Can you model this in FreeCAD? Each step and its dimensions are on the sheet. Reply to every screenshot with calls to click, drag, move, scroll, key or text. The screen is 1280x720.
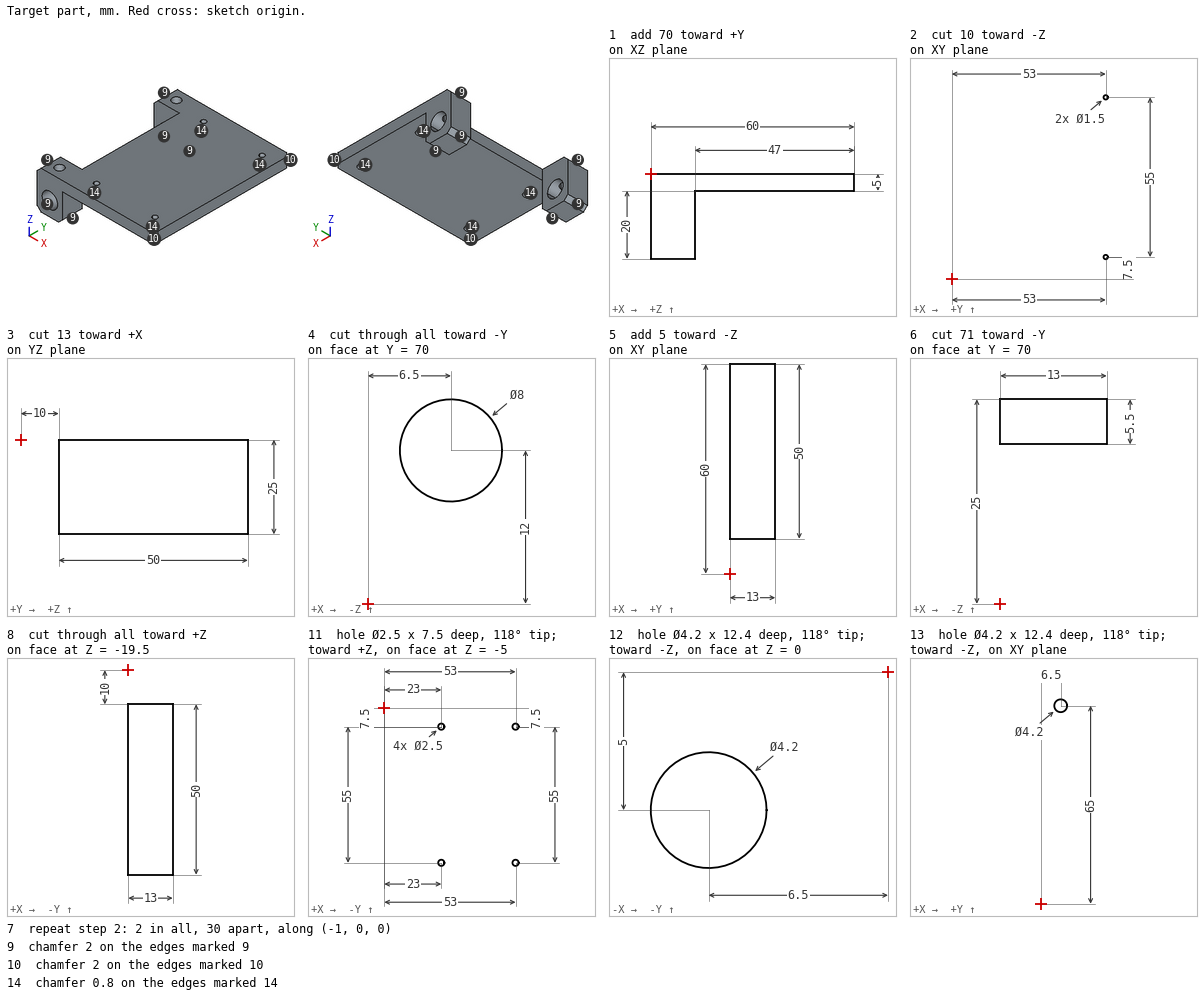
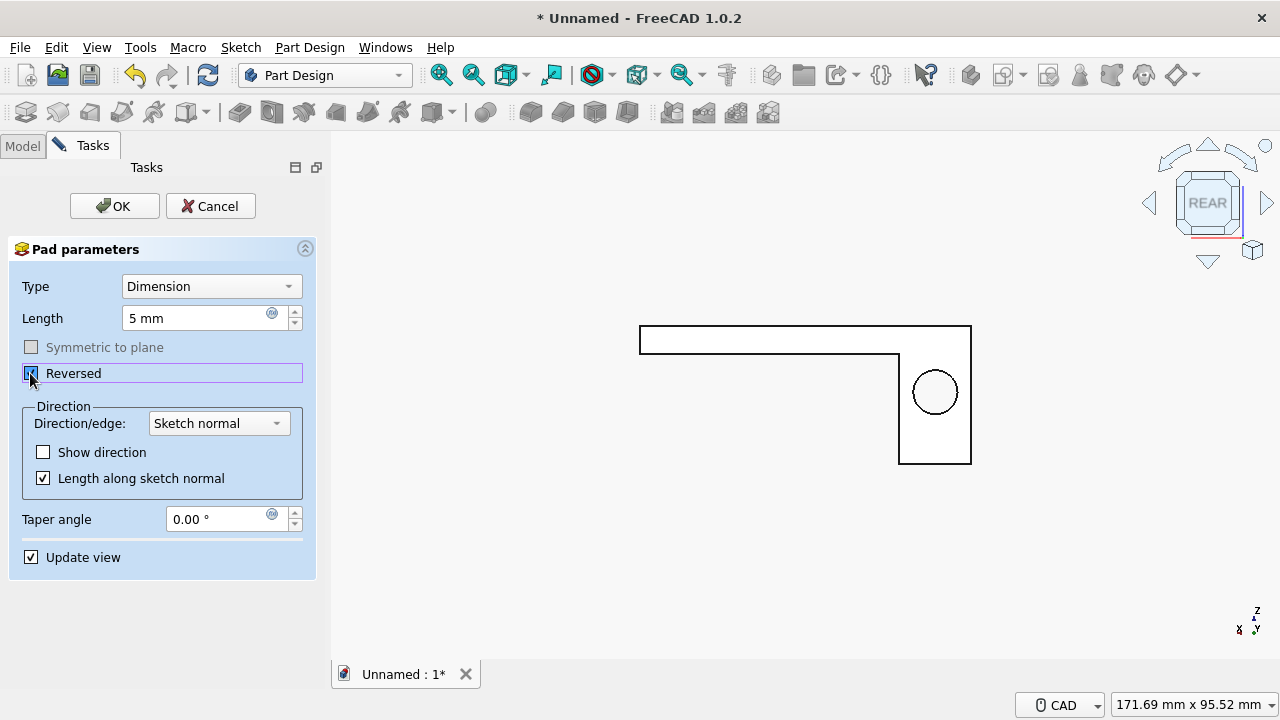
click(115, 206)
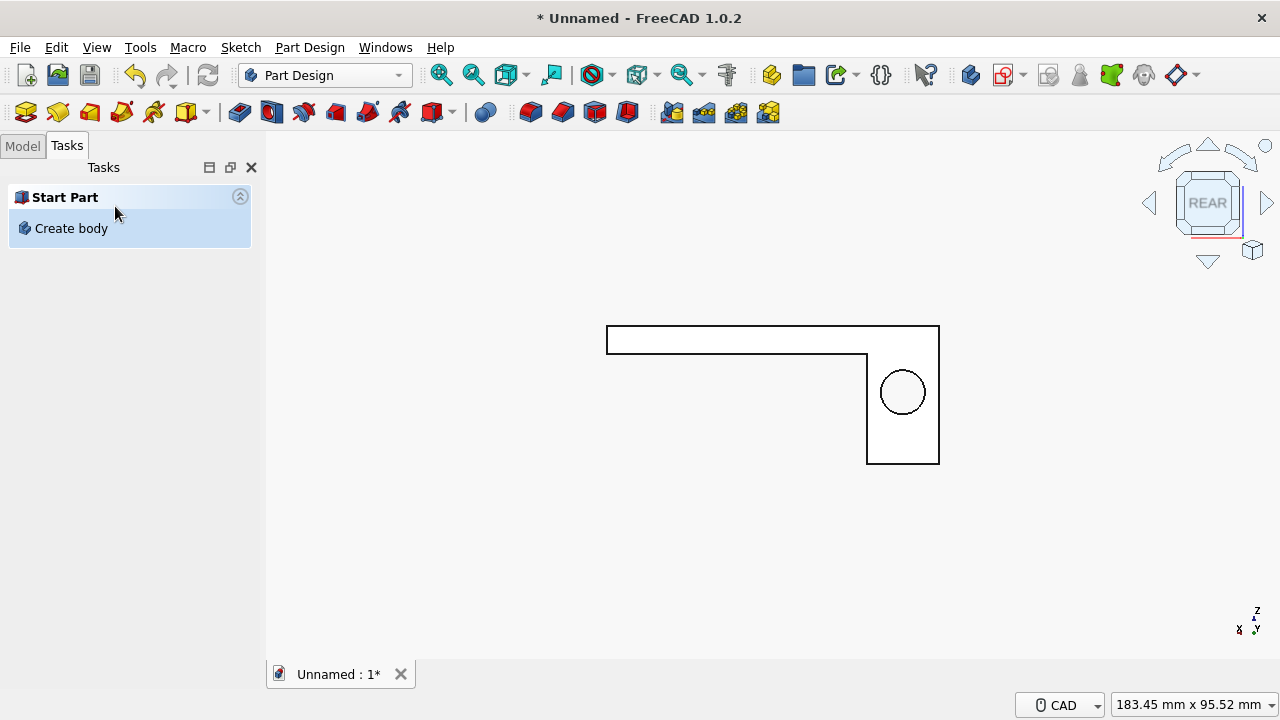
key(v)
key(f)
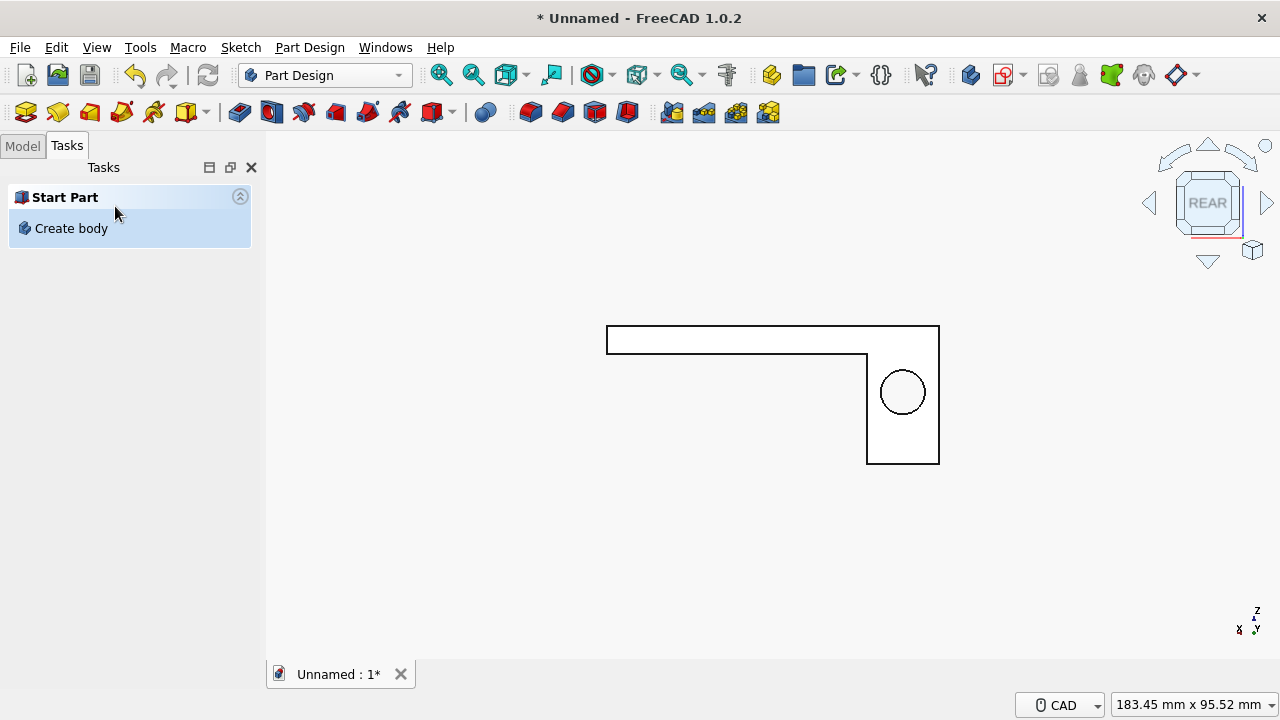
click(915, 433)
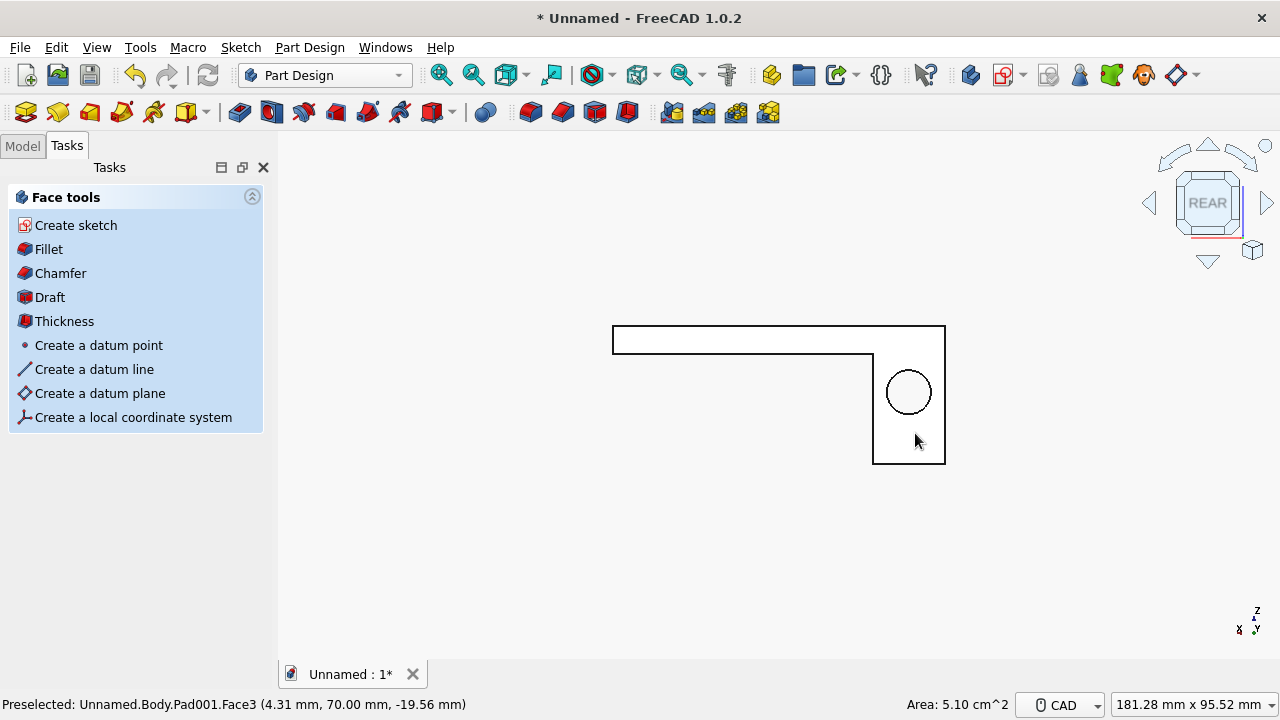
click(1004, 76)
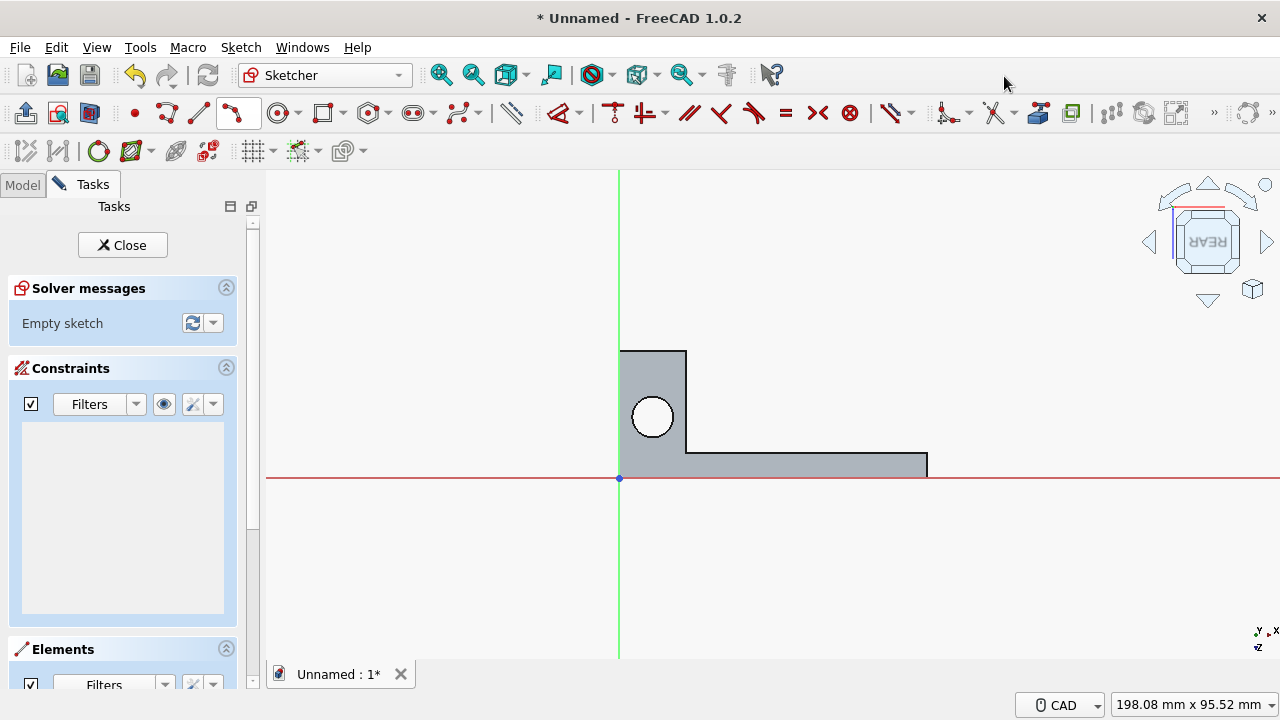
scroll(610, 414, up, 4)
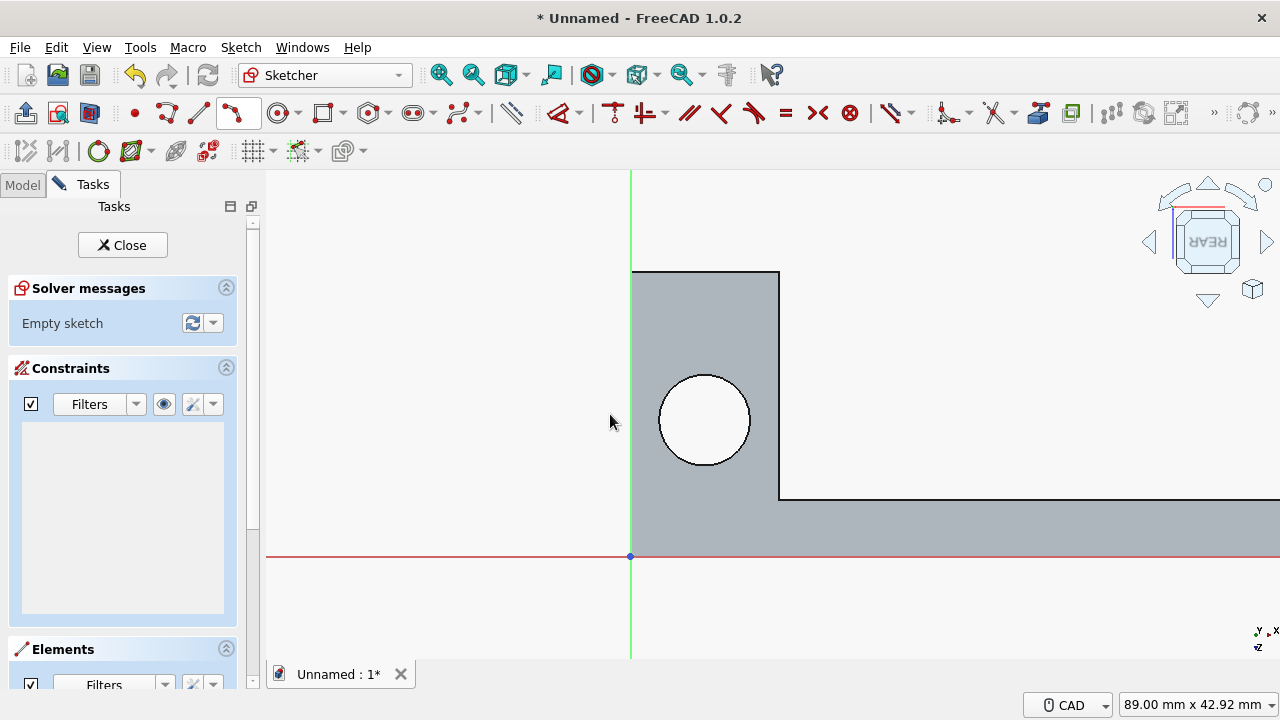
click(324, 114)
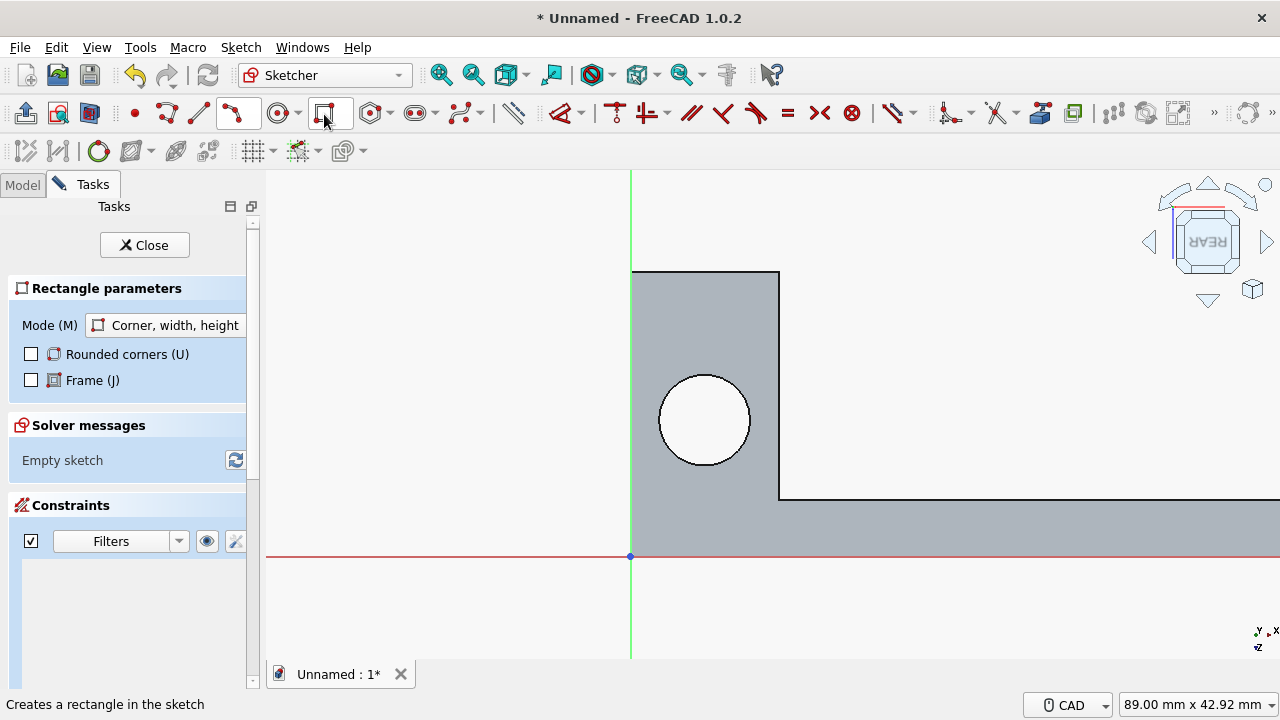
click(631, 272)
move(779, 335)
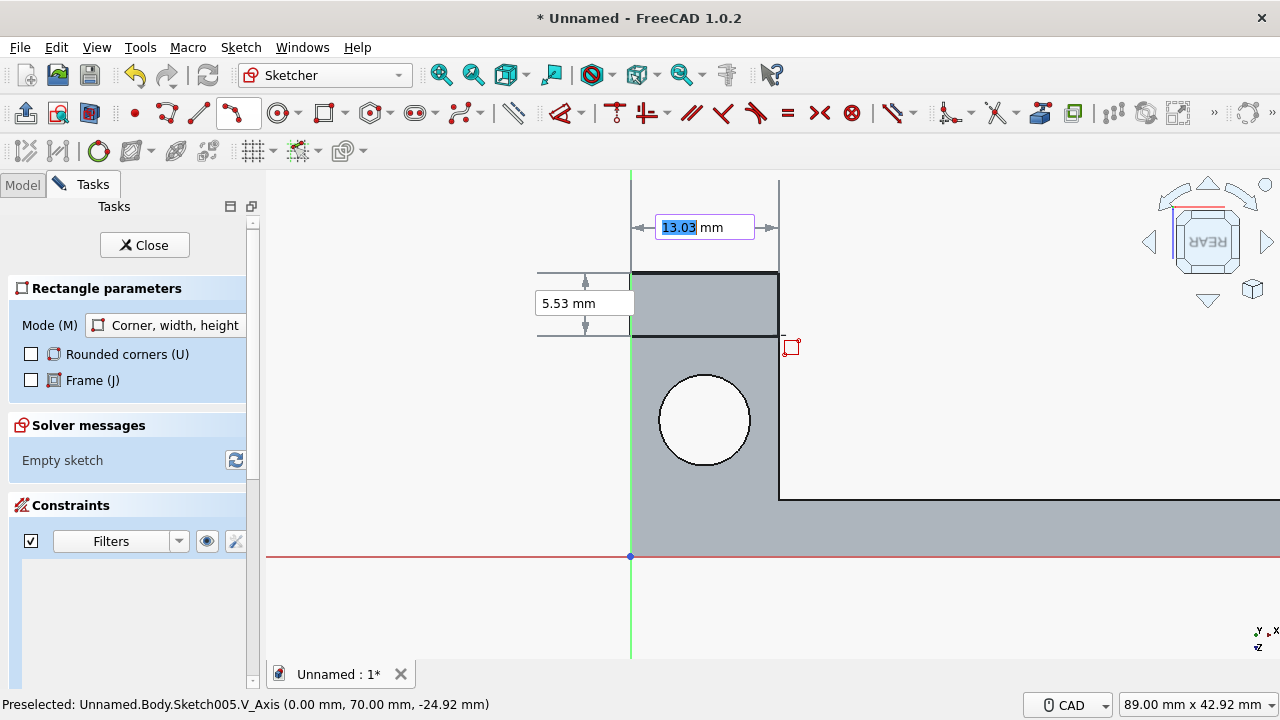
text(13)
key(Tab)
text(5.5)
key(Return)
key(Escape)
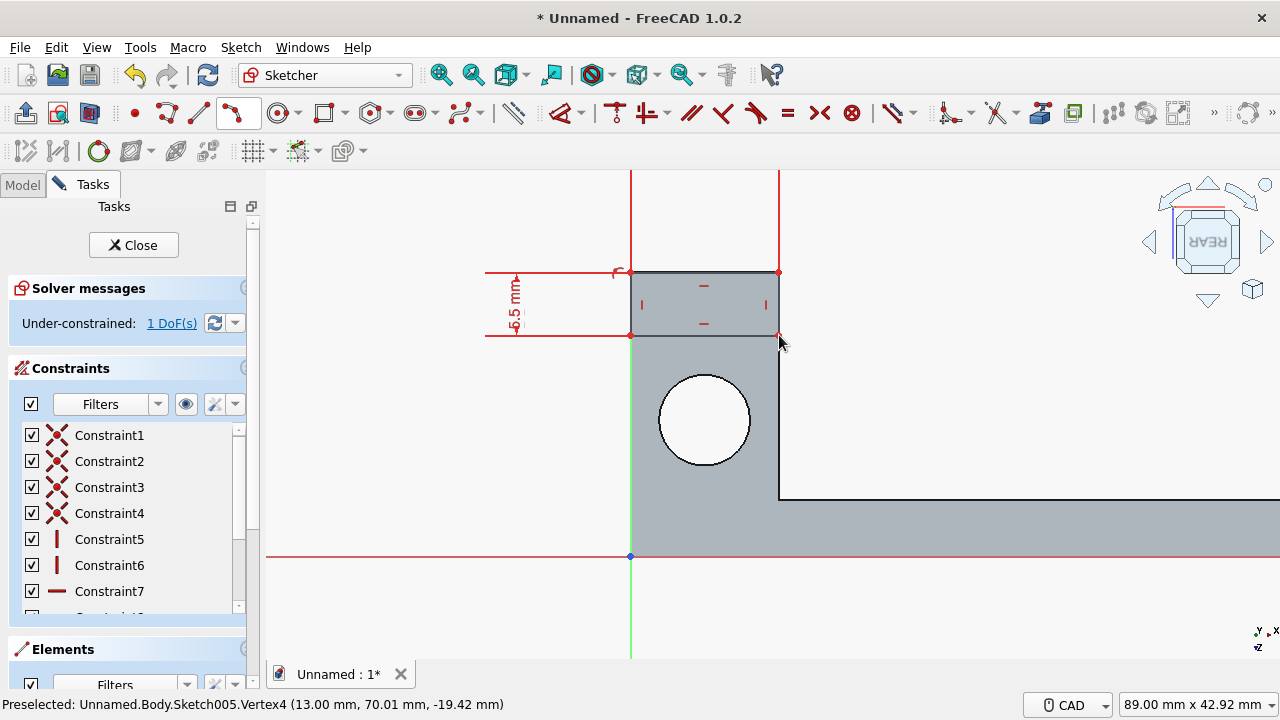
key(d)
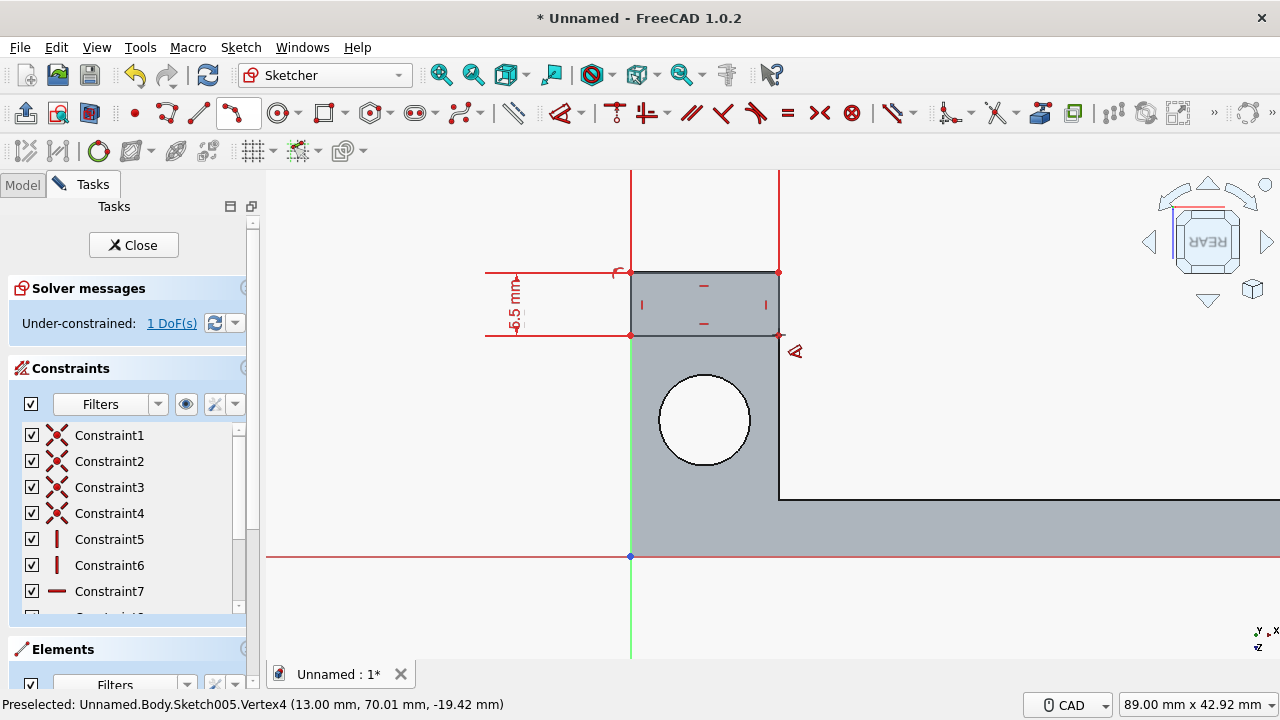
click(631, 273)
click(597, 415)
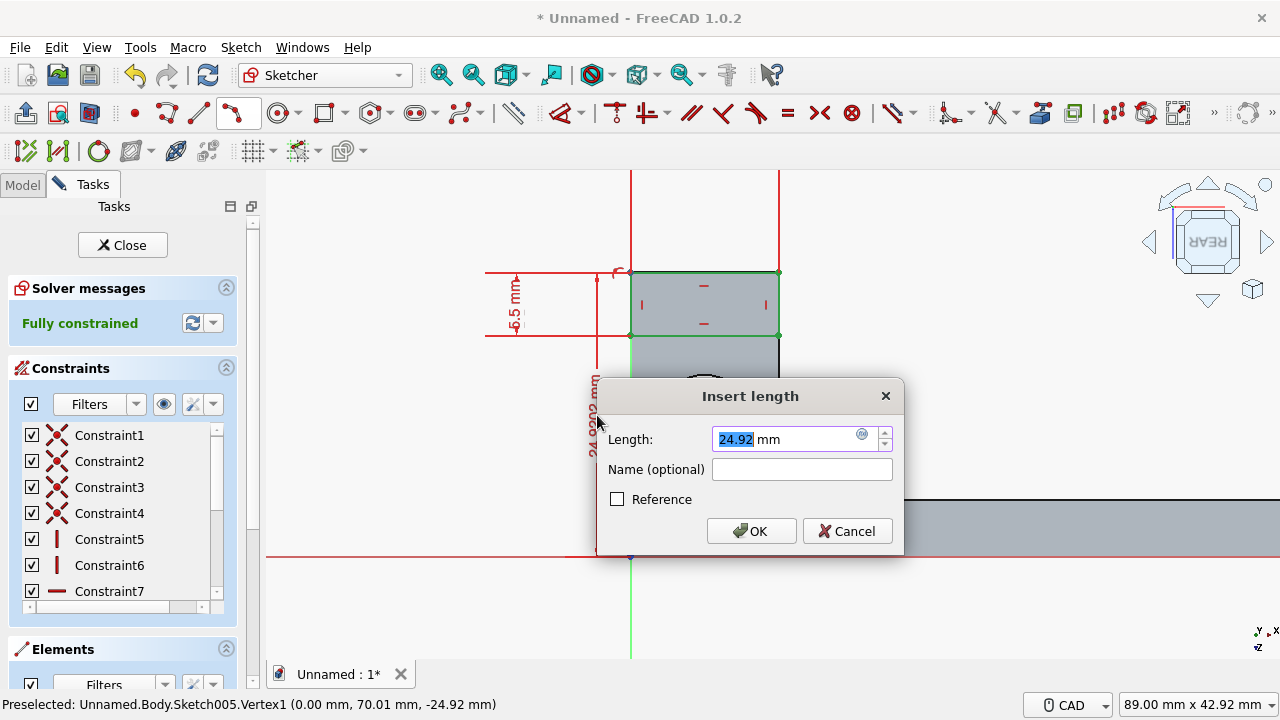
text(25)
key(Return)
key(Escape)